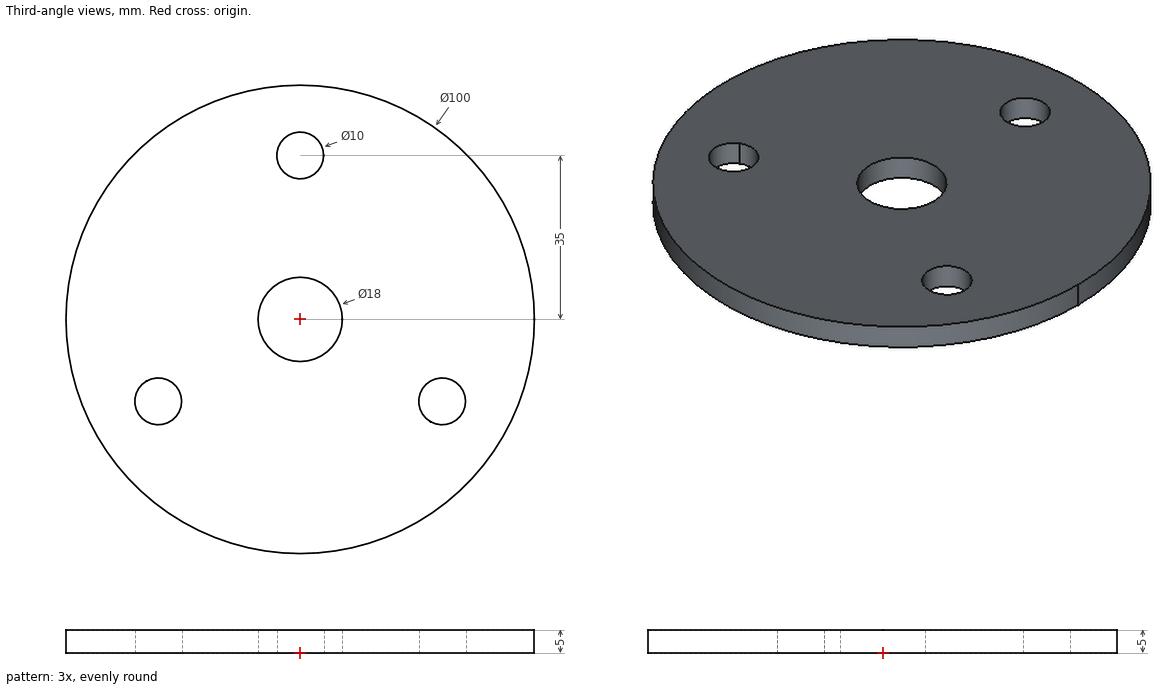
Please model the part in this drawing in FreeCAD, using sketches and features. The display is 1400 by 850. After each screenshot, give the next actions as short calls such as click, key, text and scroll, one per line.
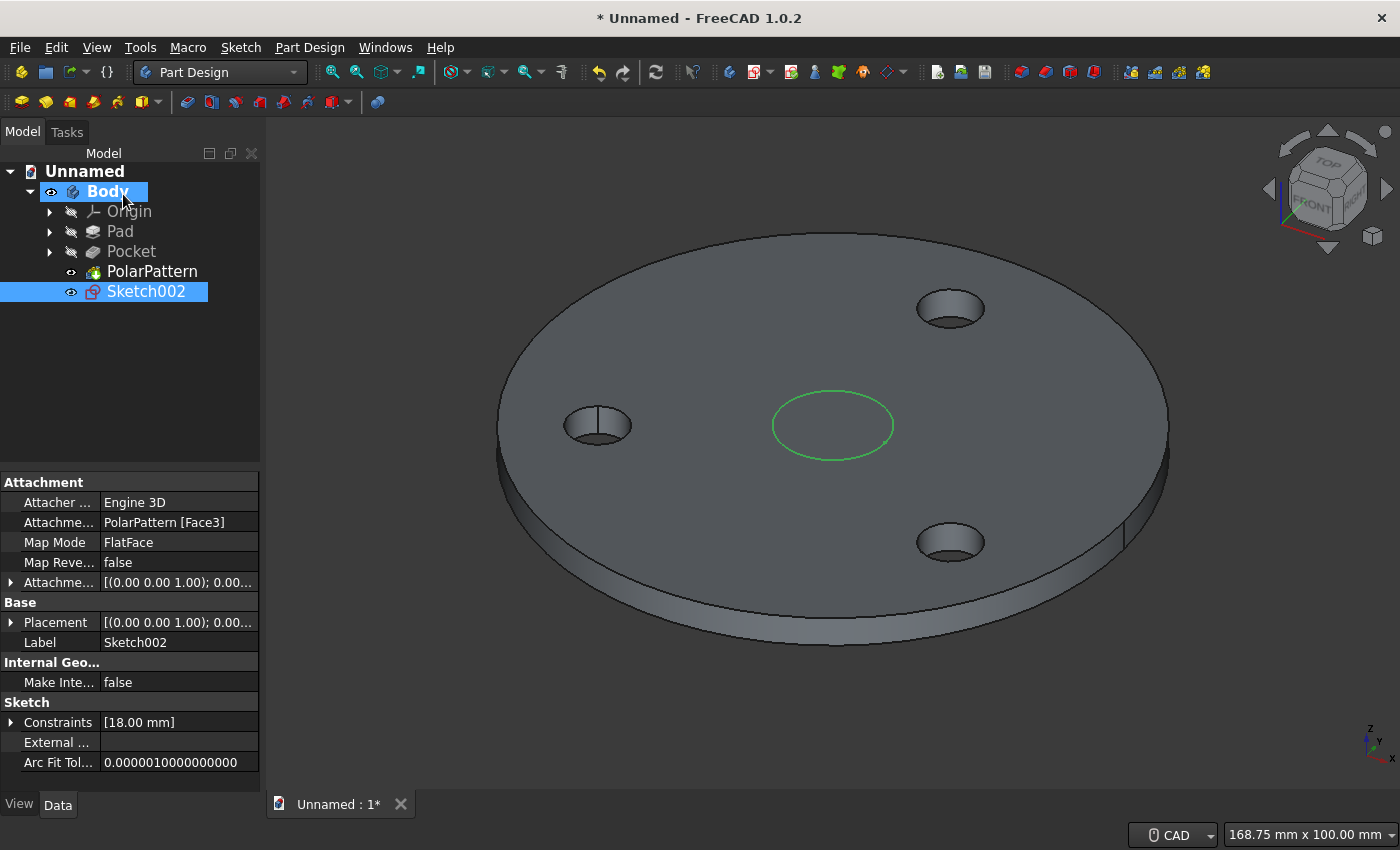
click(188, 102)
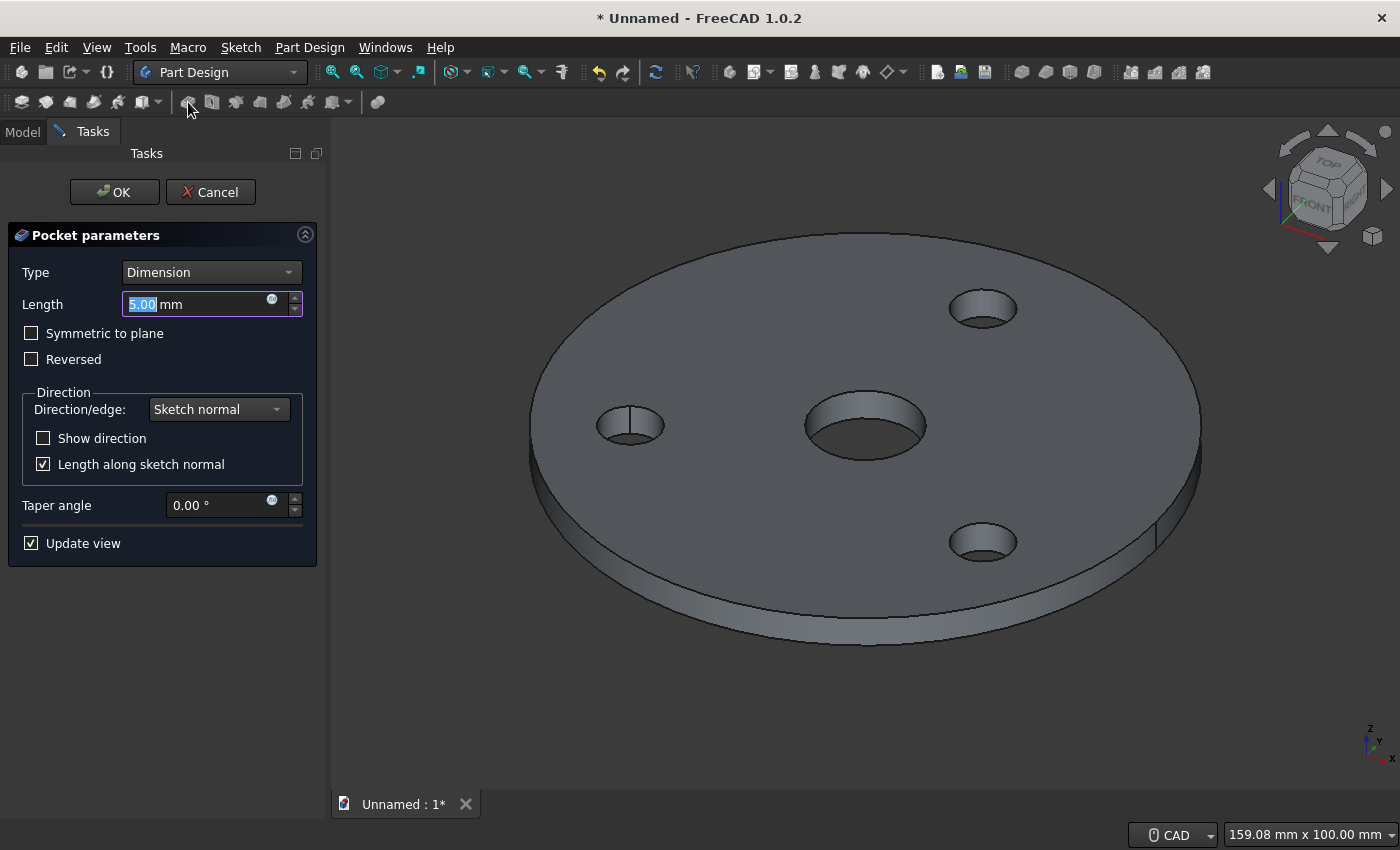
text(5)
key(Tab)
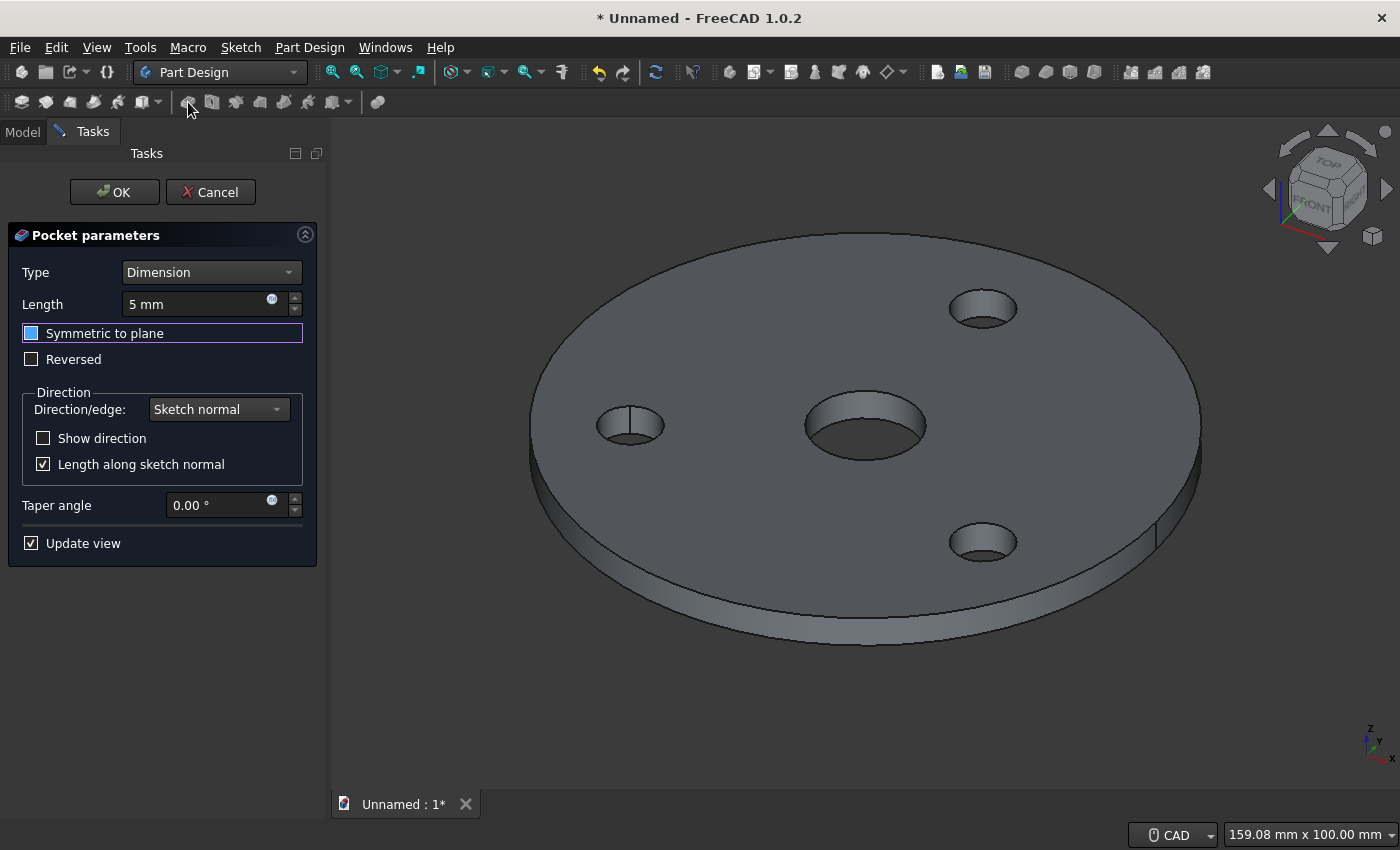
click(115, 192)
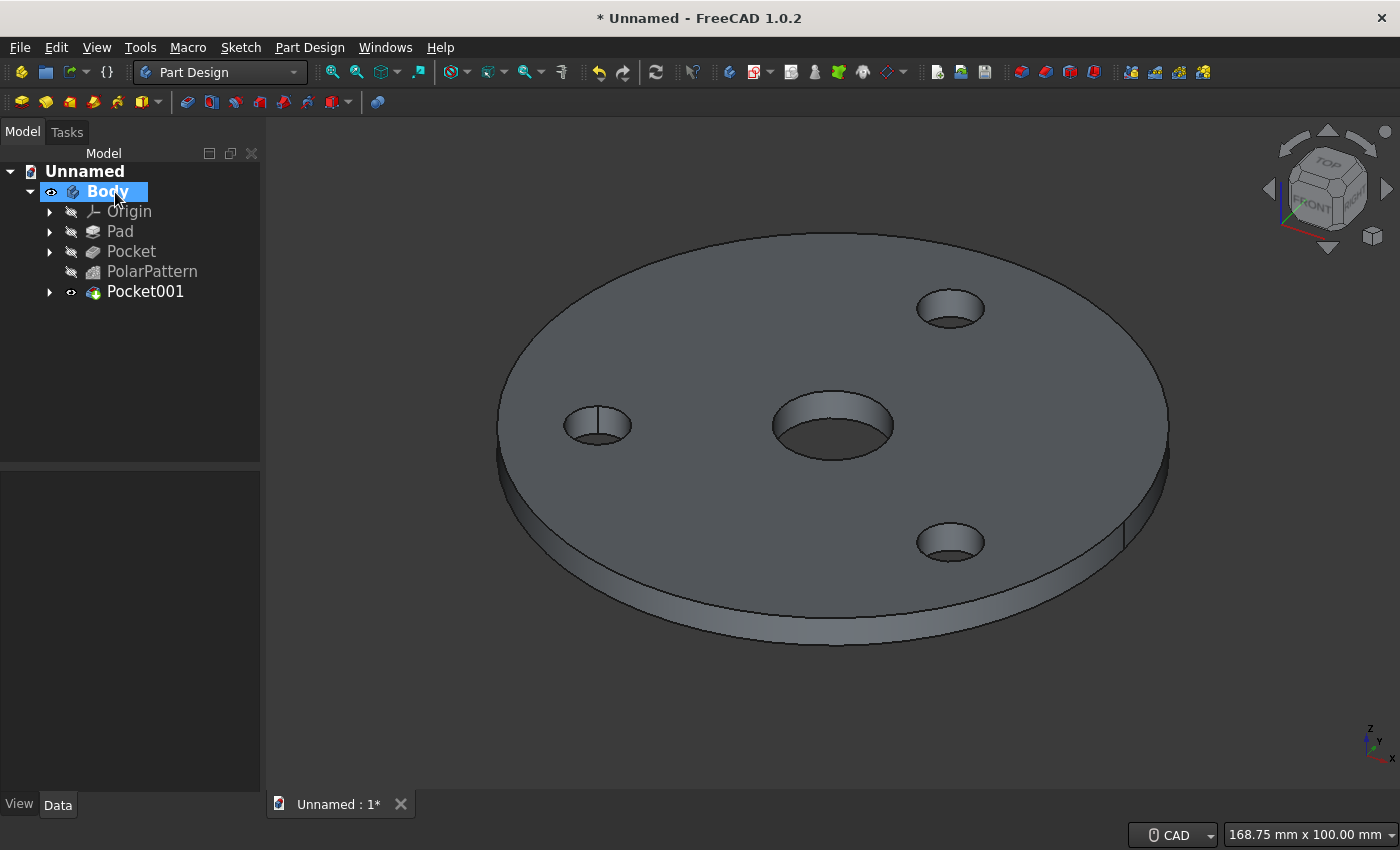
key(0)